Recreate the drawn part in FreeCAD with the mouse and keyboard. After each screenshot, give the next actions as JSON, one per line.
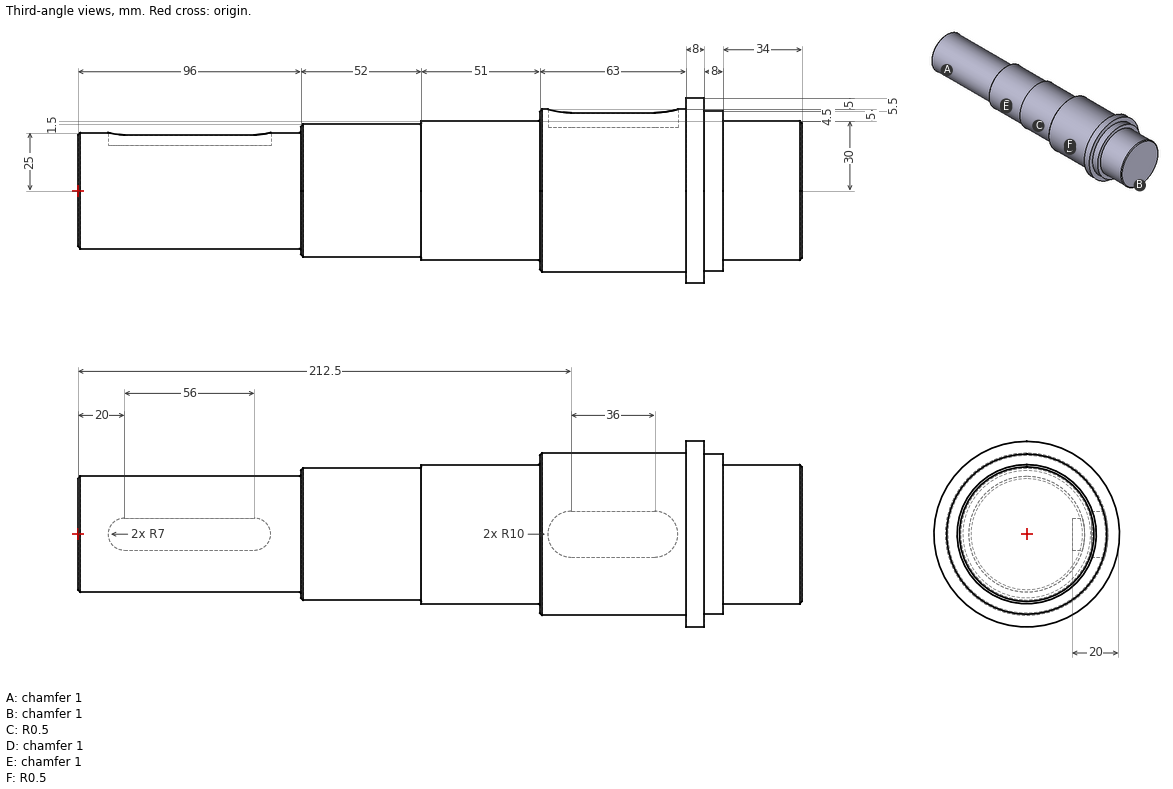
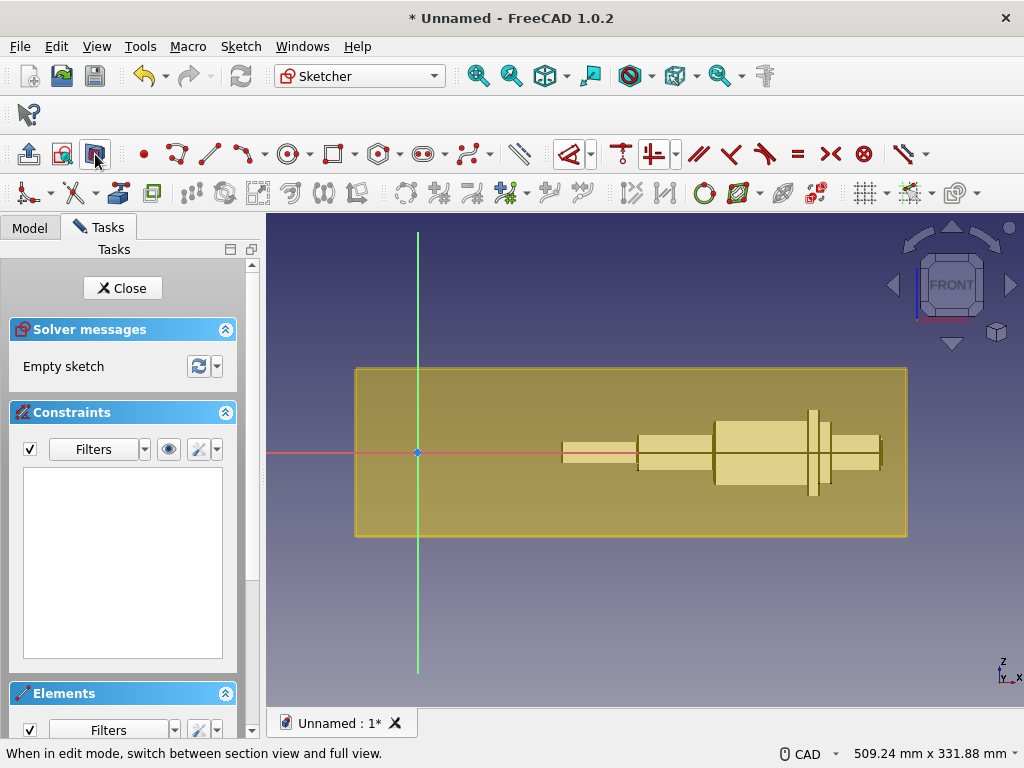
{"action": "scroll", "coordinate": [807, 451], "scroll_direction": "up", "scroll_amount": 8}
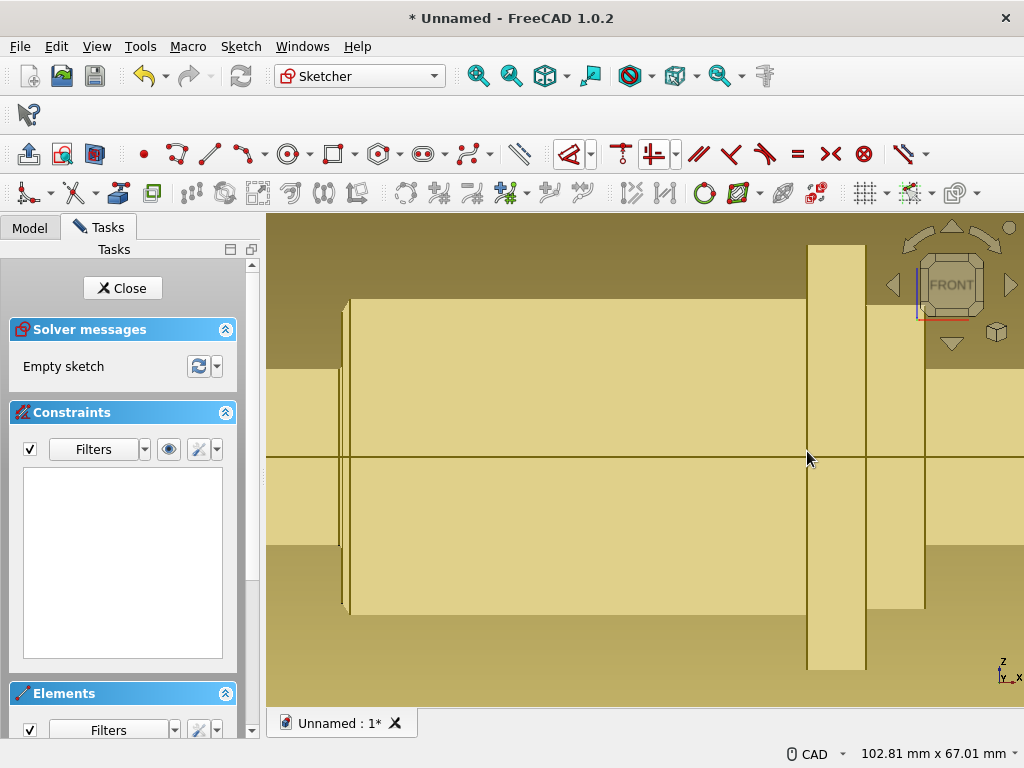
{"action": "key", "text": "g s"}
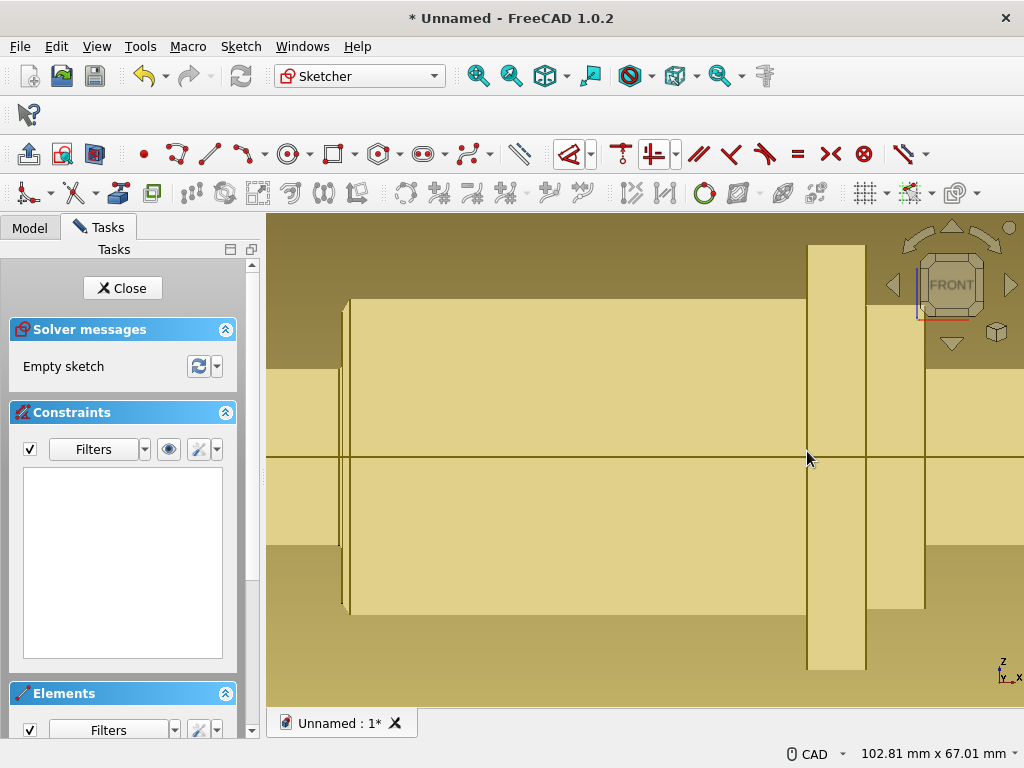
{"action": "left_click", "coordinate": [442, 457]}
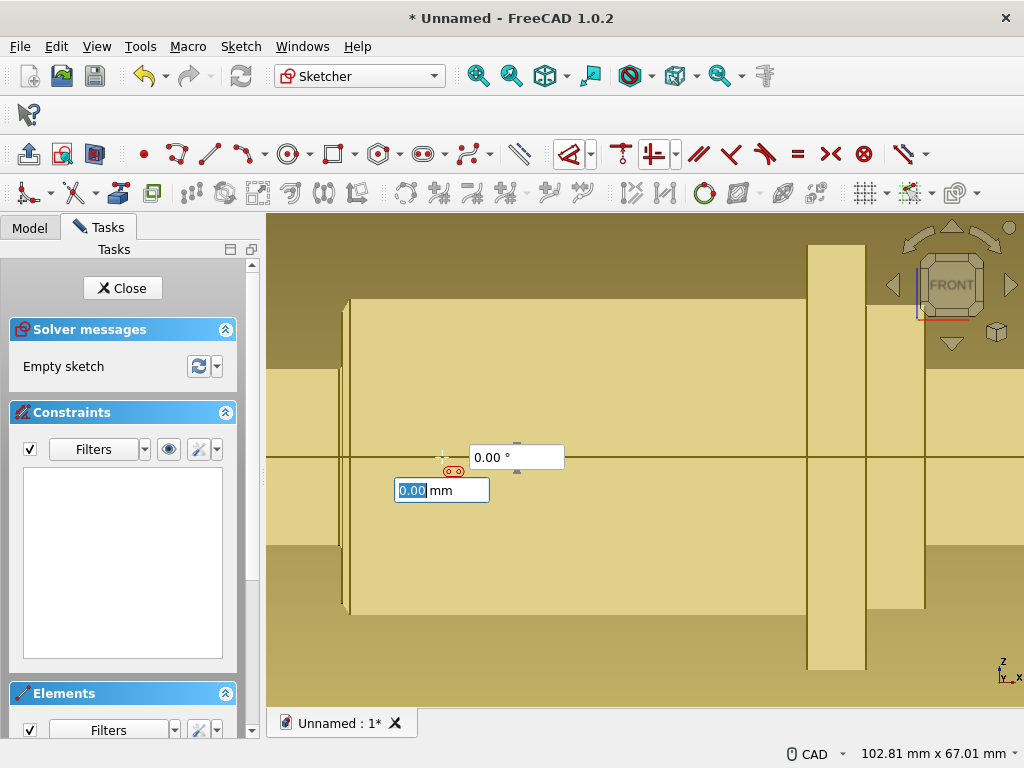
{"action": "left_click", "coordinate": [707, 448]}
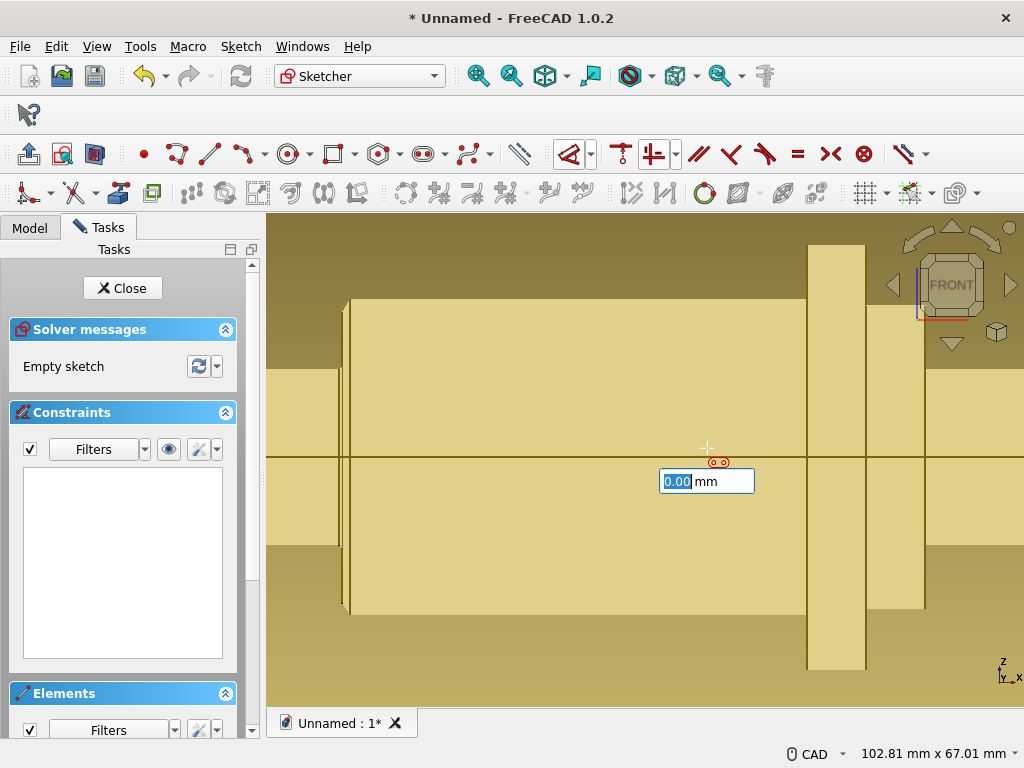
{"action": "left_click", "coordinate": [575, 531]}
{"action": "key", "text": "Escape"}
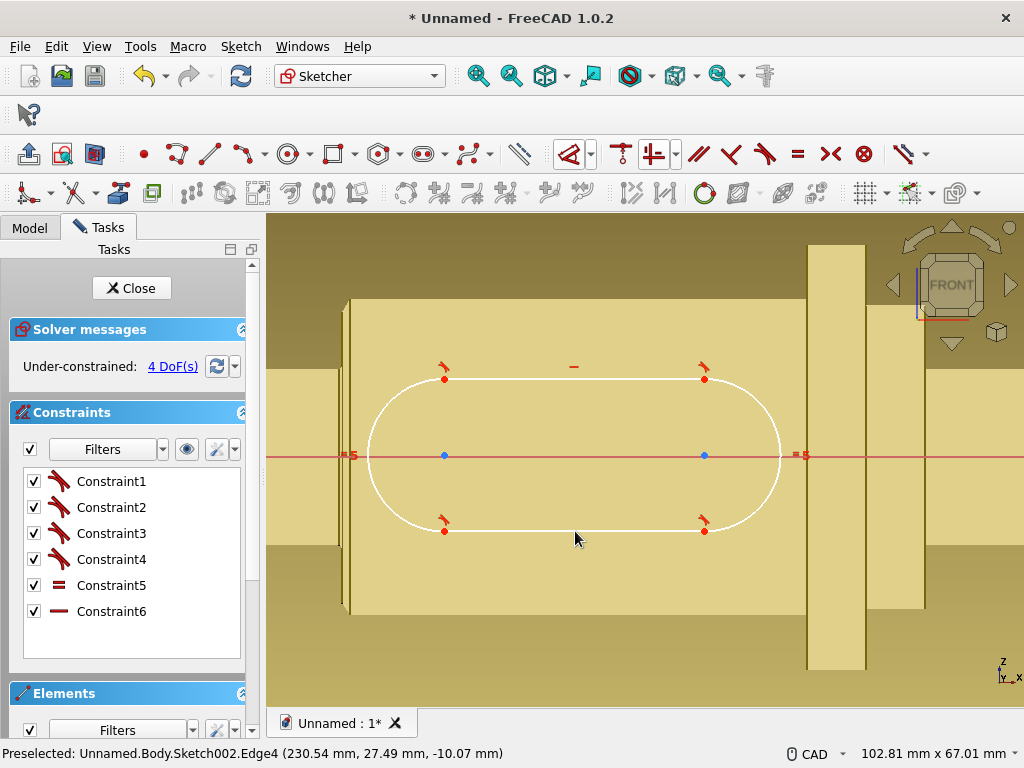
{"action": "left_click", "coordinate": [444, 455]}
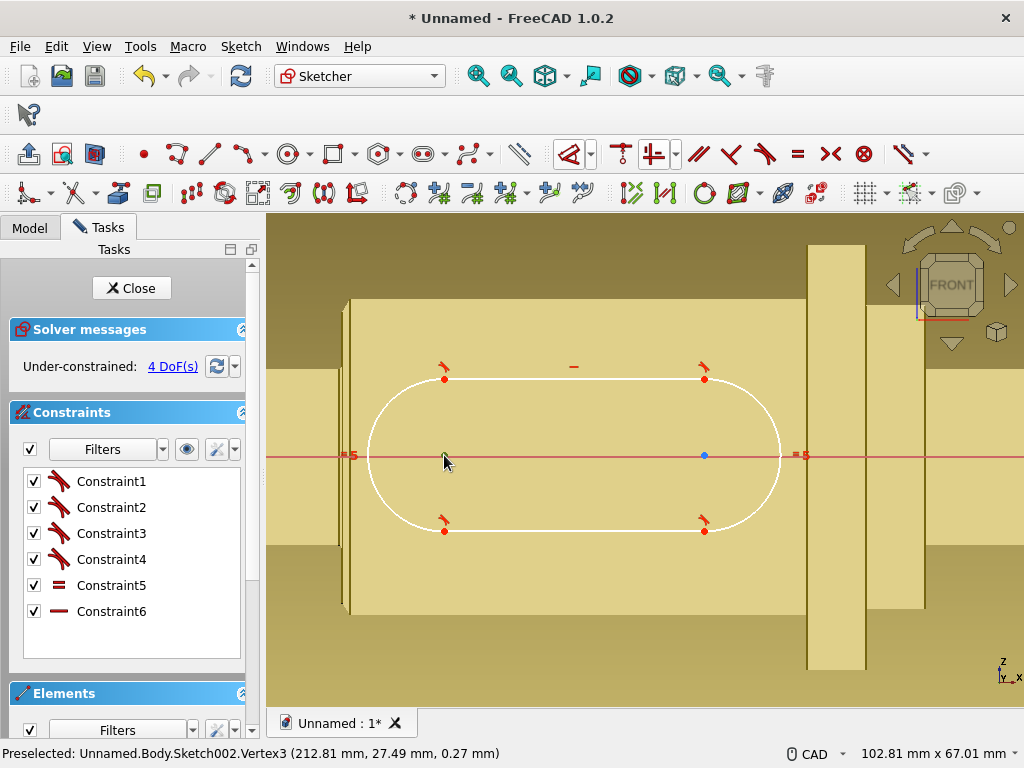
{"action": "left_click", "coordinate": [334, 457]}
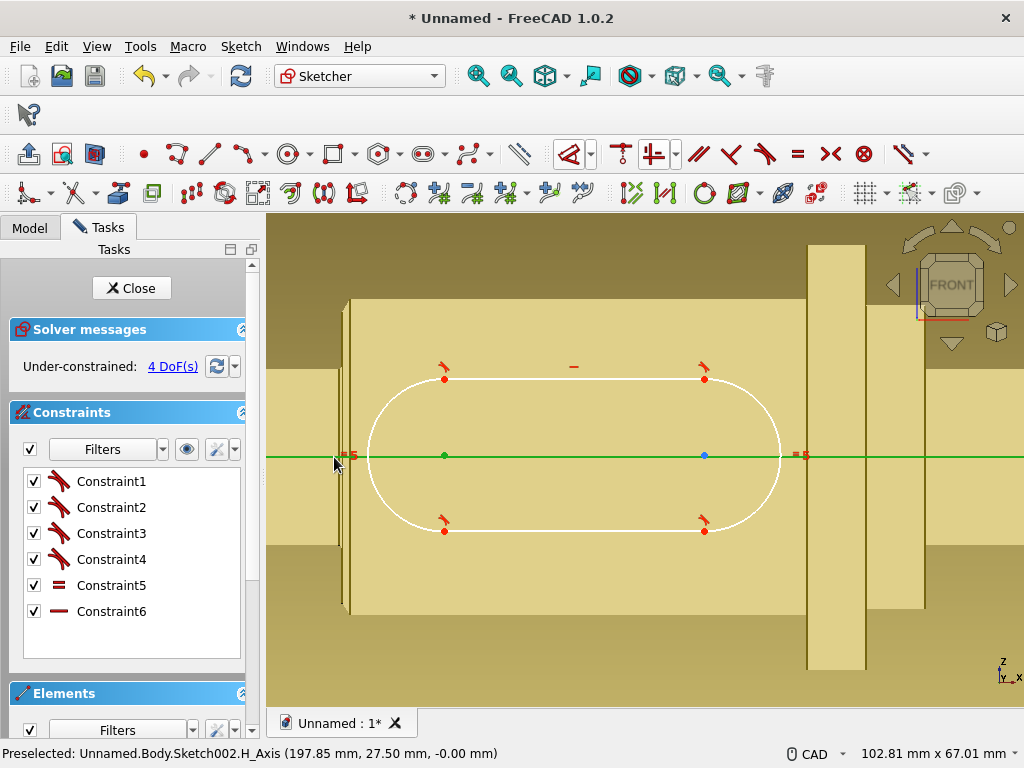
{"action": "key", "text": "c"}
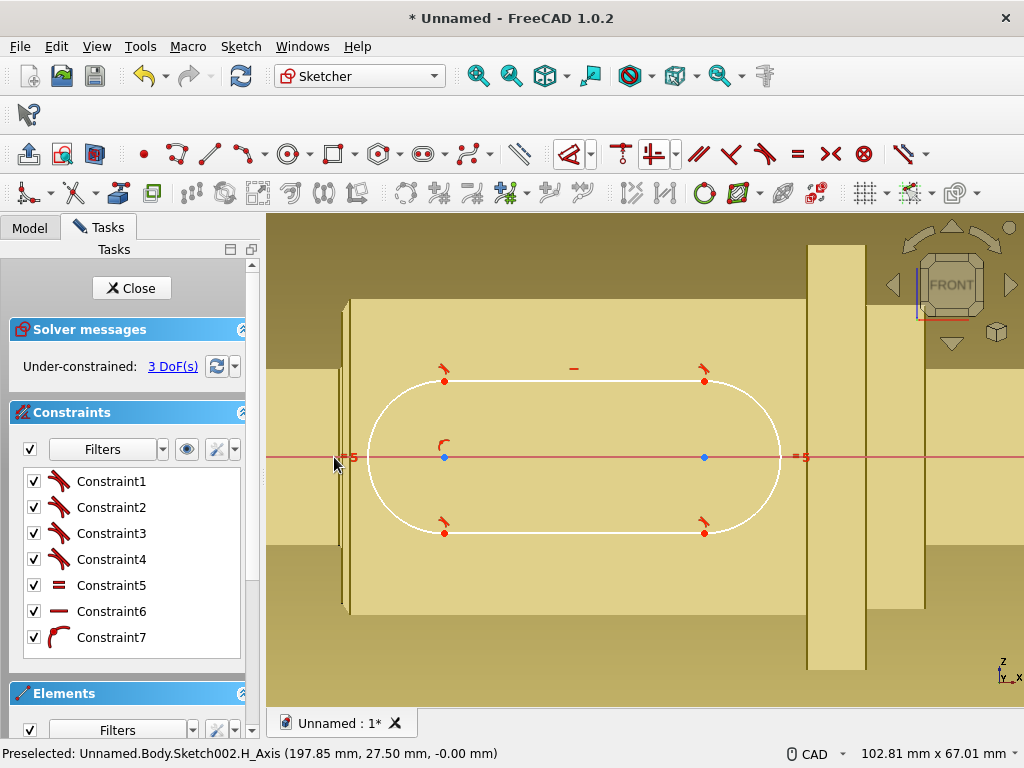
{"action": "left_click", "coordinate": [383, 412]}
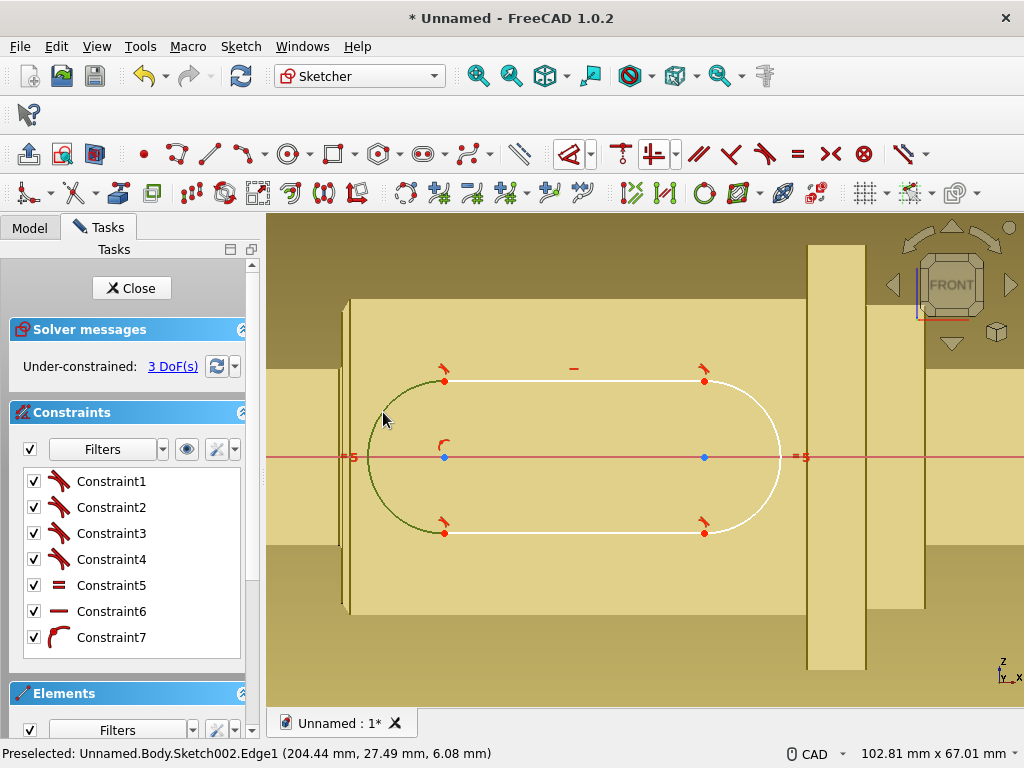
{"action": "left_click", "coordinate": [590, 154]}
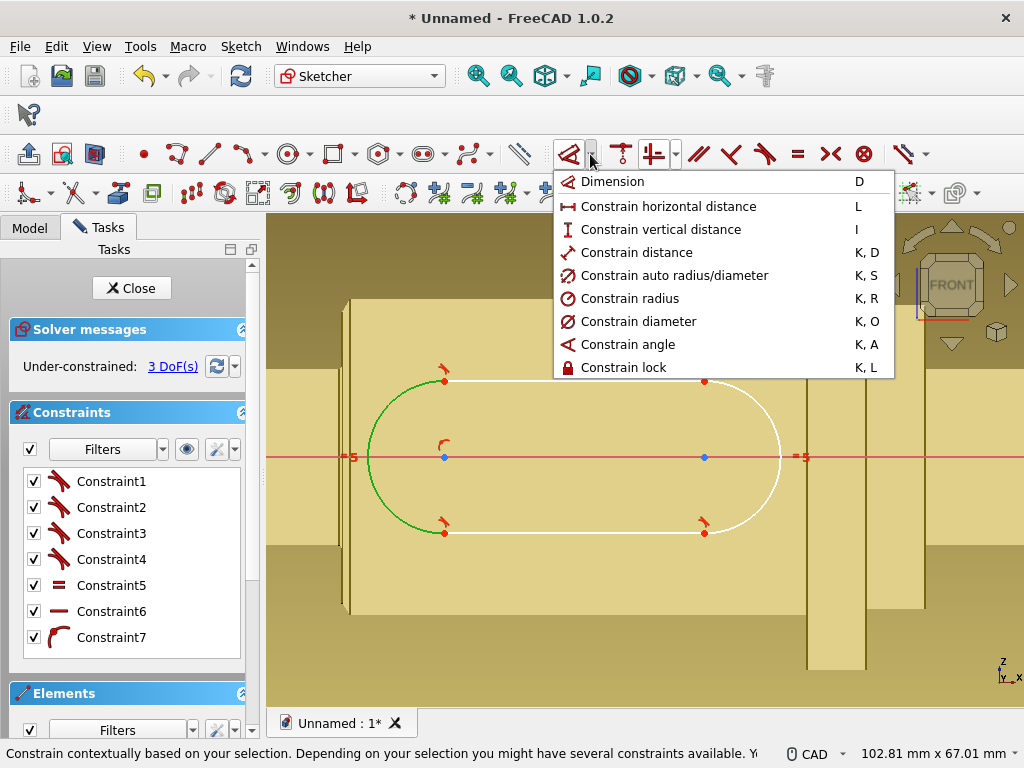
{"action": "left_click", "coordinate": [724, 298]}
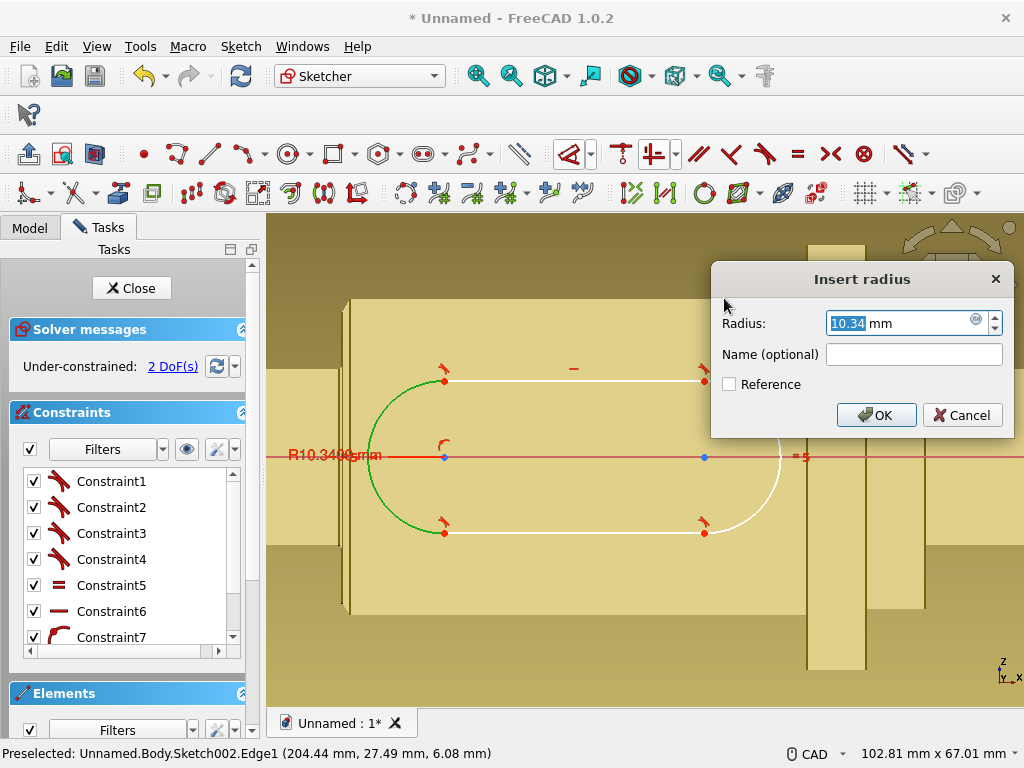
{"action": "type", "text": "10"}
{"action": "key", "text": "Return"}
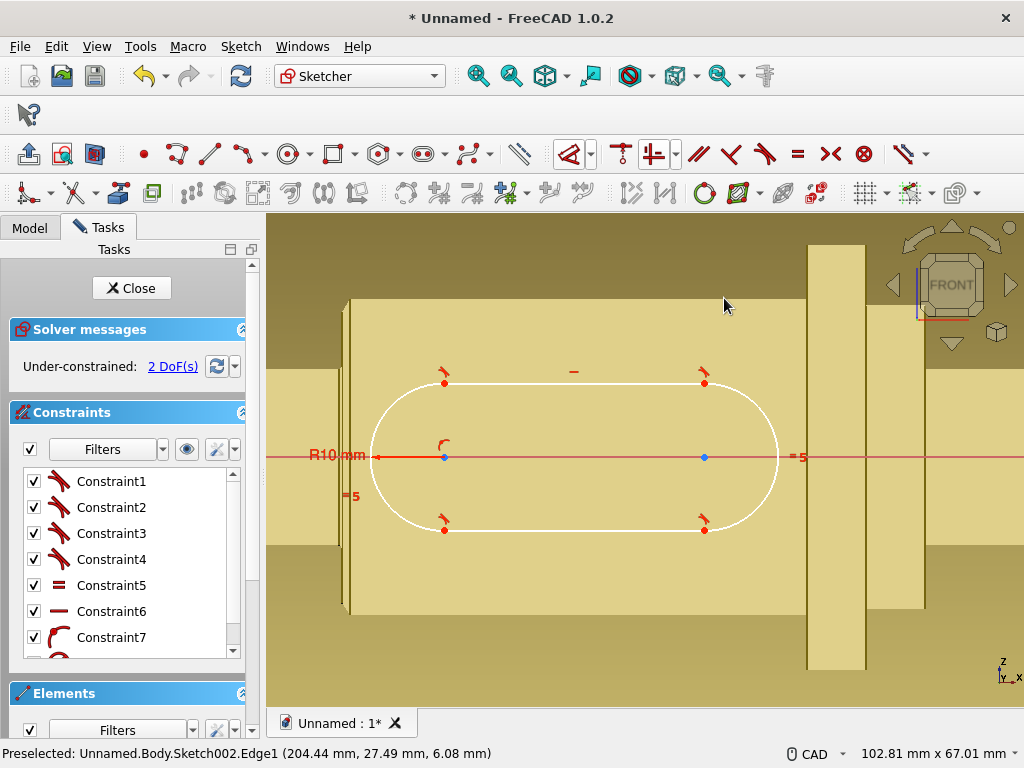
{"action": "left_click", "coordinate": [522, 384]}